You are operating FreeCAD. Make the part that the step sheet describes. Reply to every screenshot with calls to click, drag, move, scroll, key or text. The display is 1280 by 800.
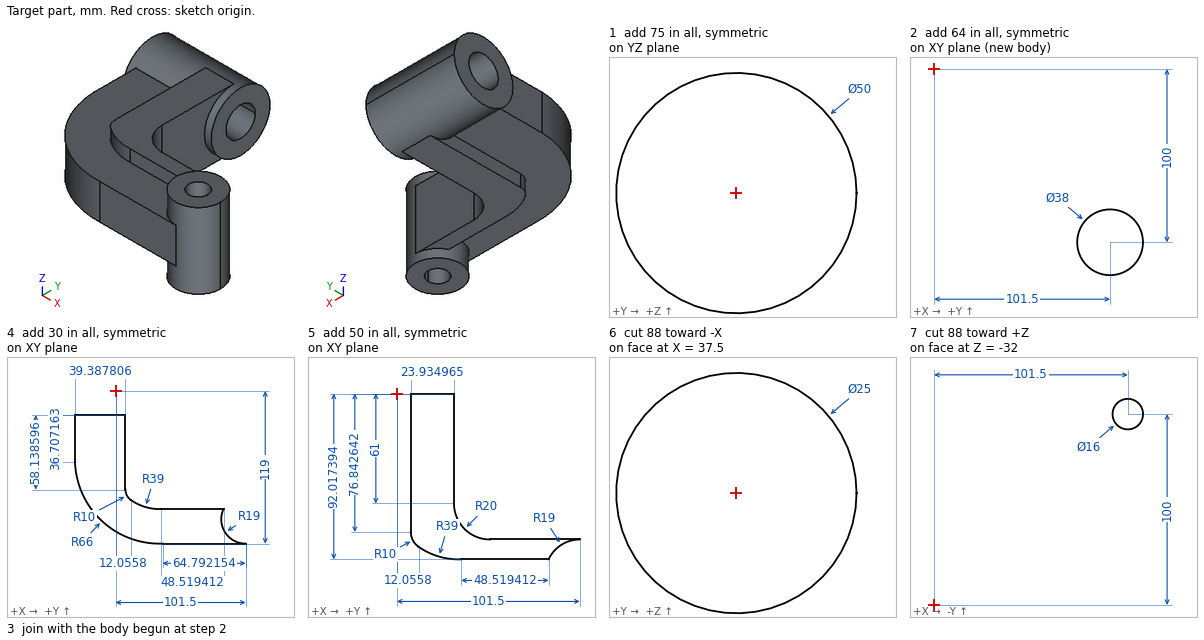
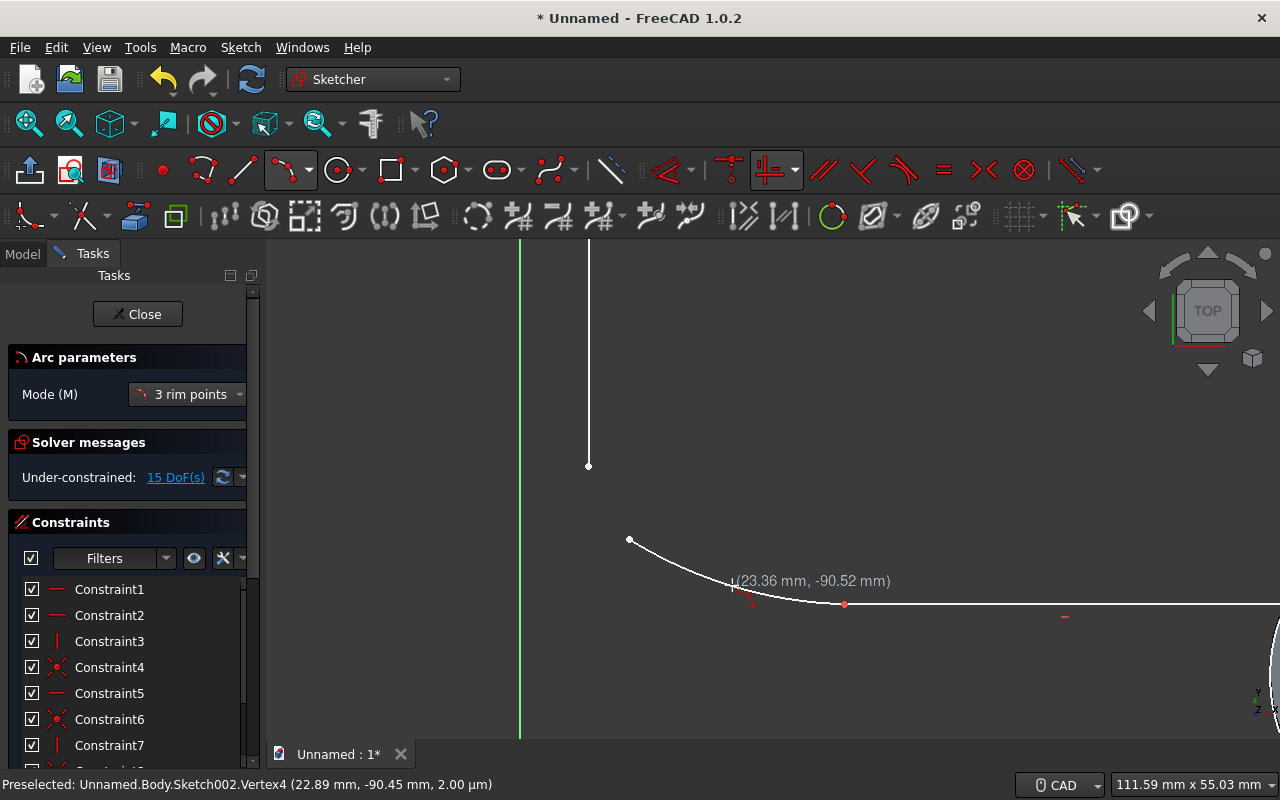
scroll(647, 569, down, 6)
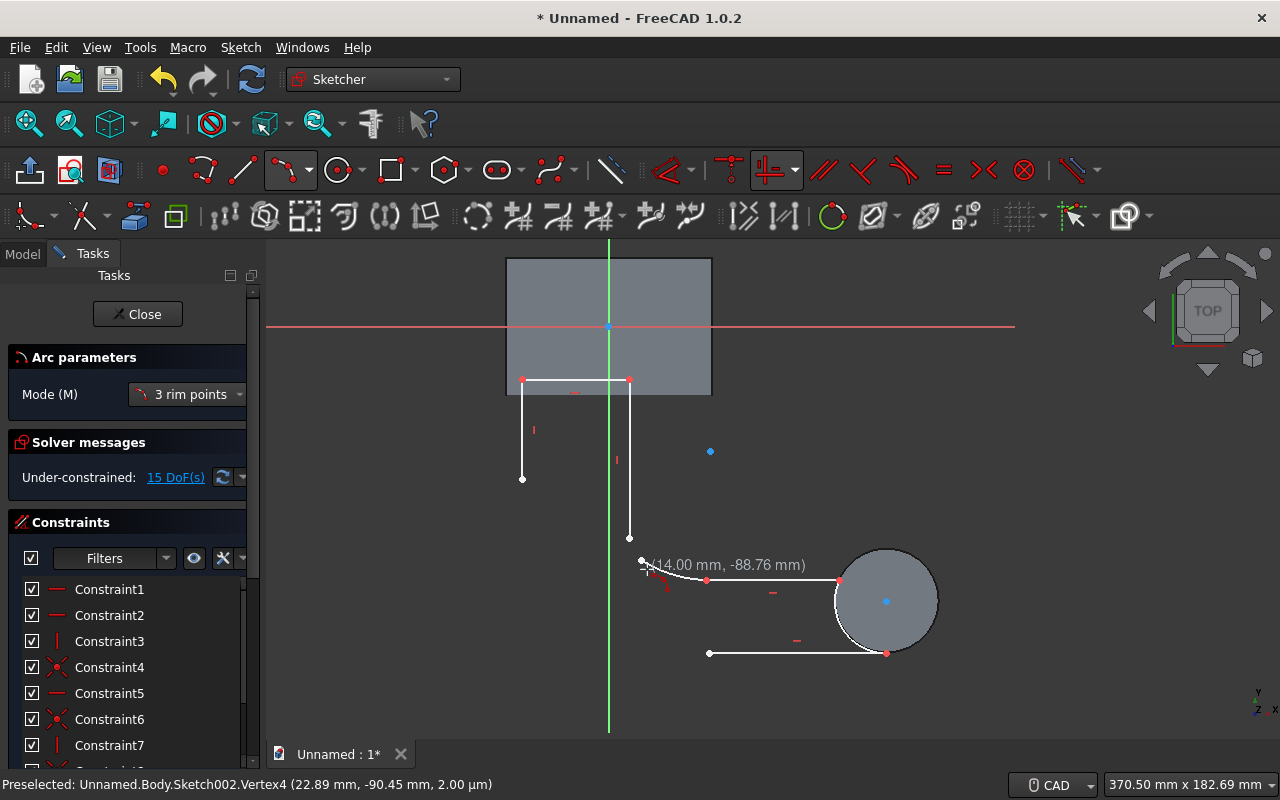
click(642, 561)
click(630, 539)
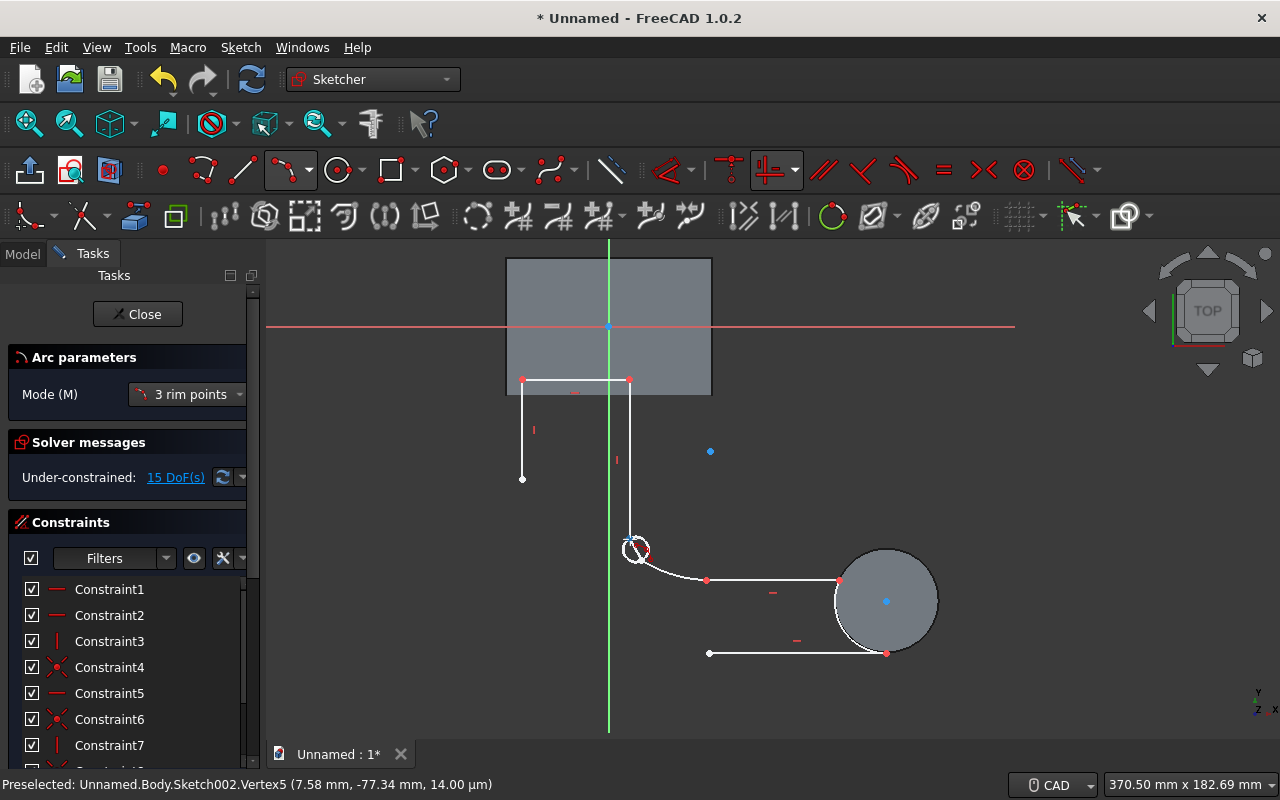
scroll(633, 550, up, 9)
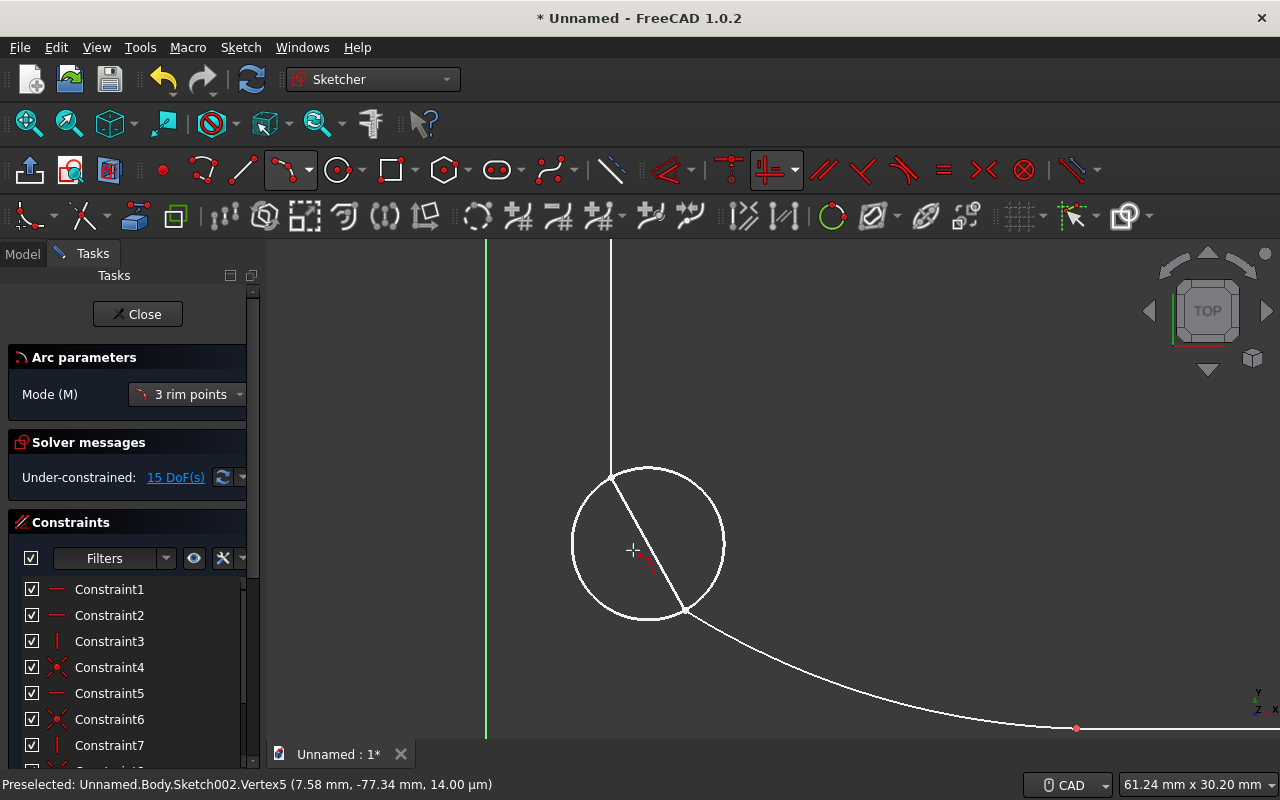
click(633, 546)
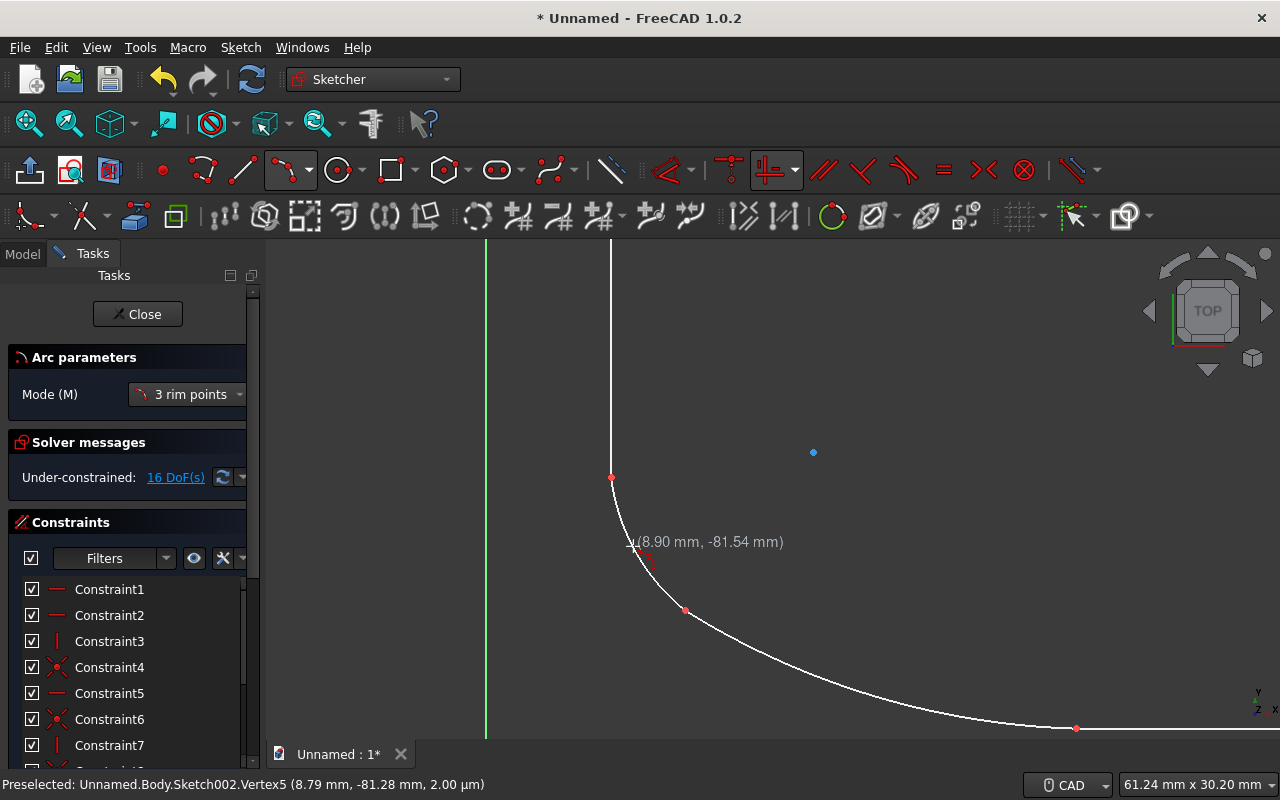
scroll(633, 550, down, 9)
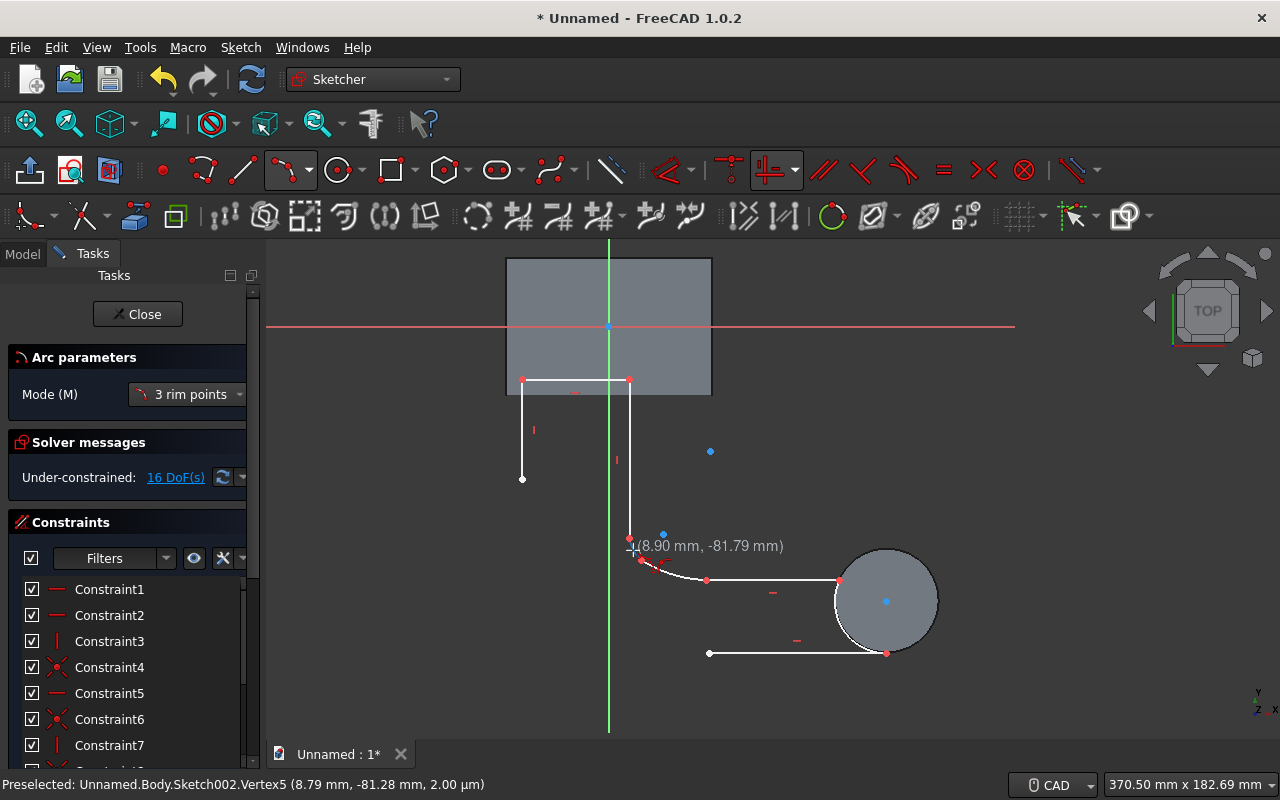
click(522, 480)
click(709, 653)
click(580, 604)
key(Escape)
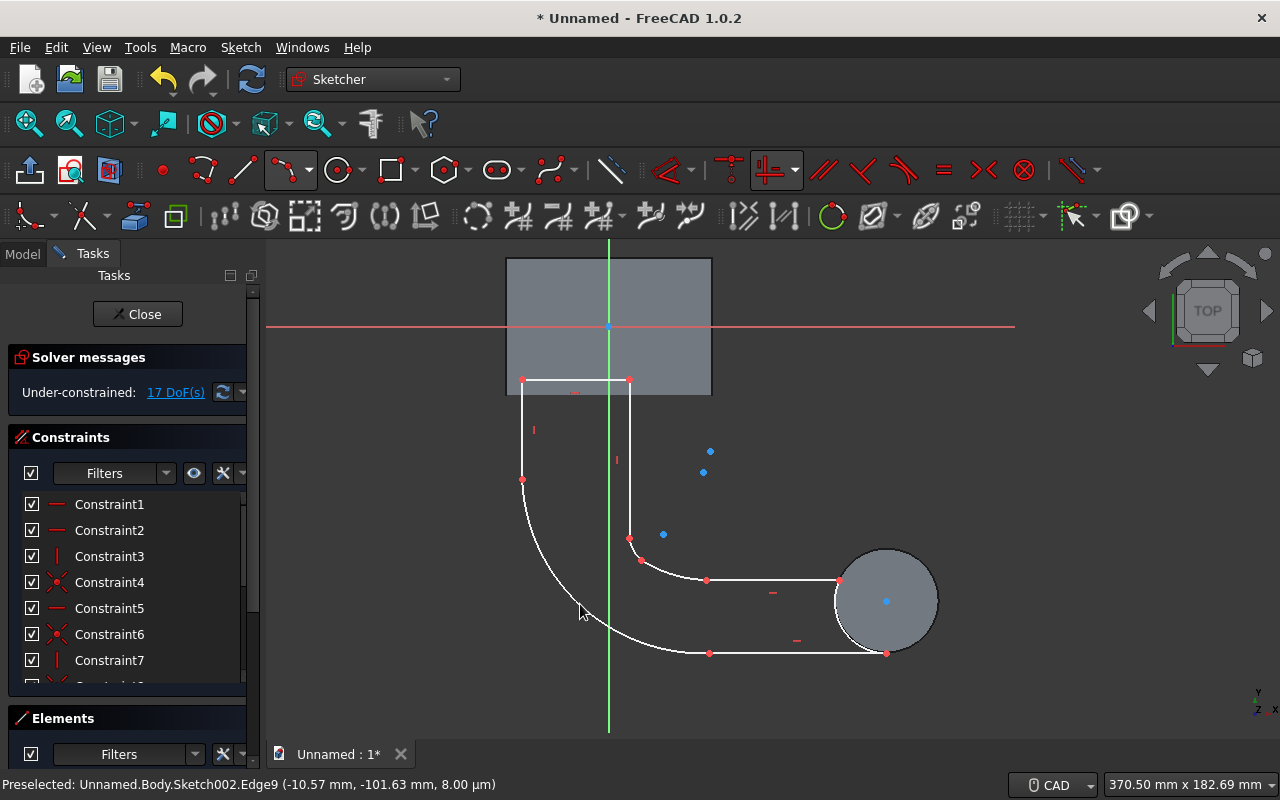
click(762, 653)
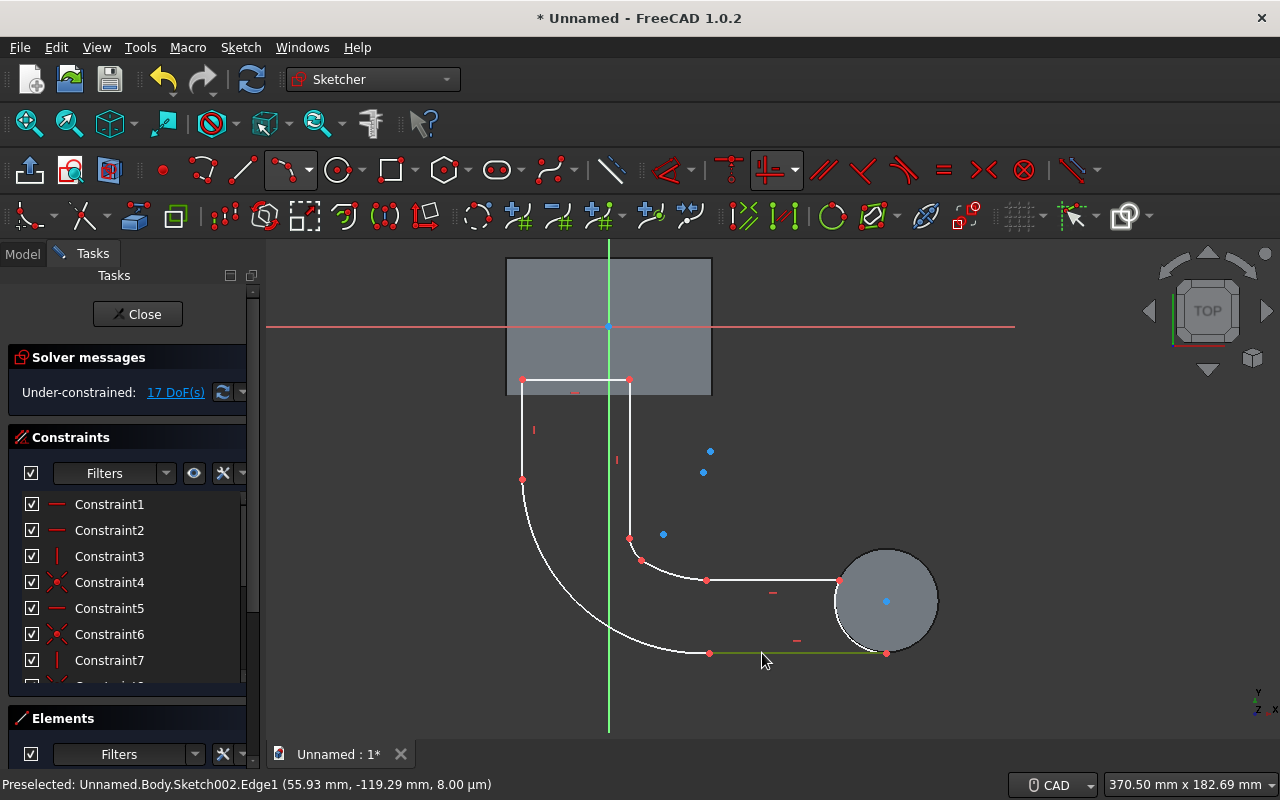
click(836, 610)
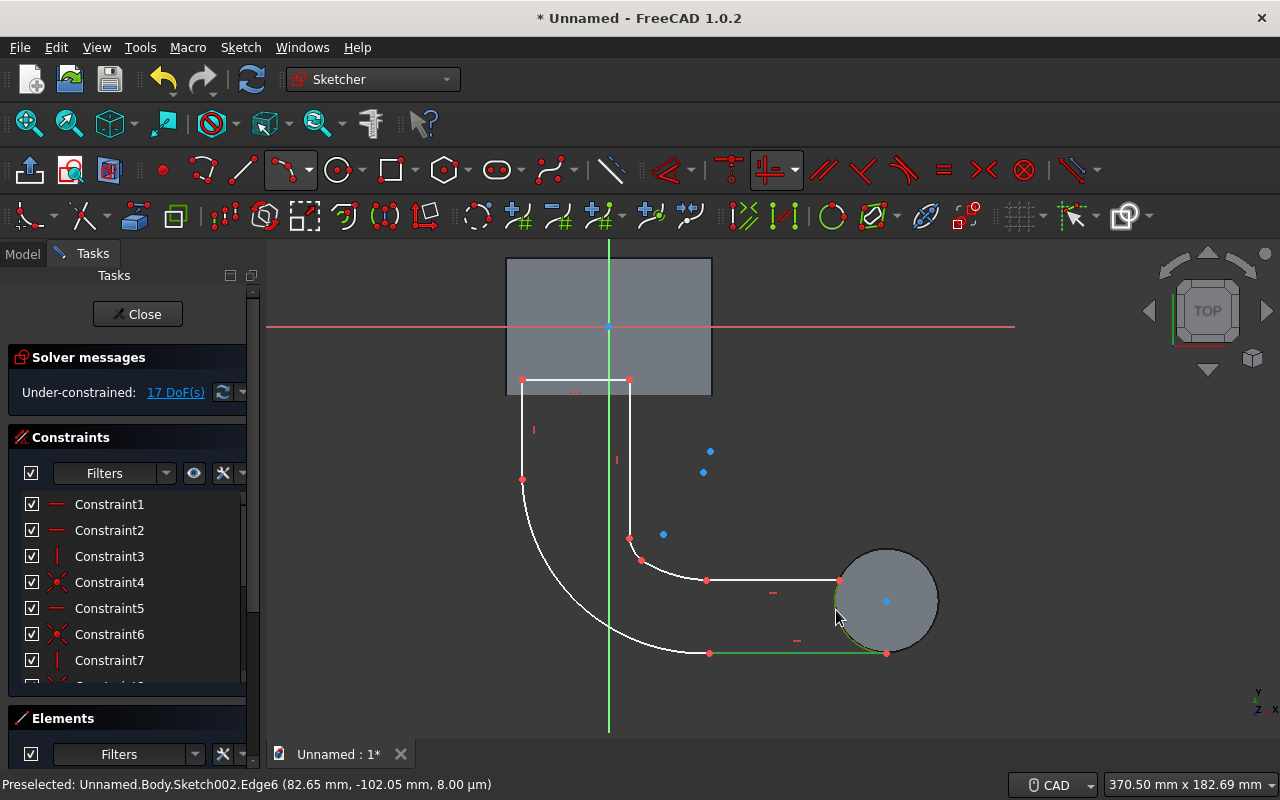
click(904, 170)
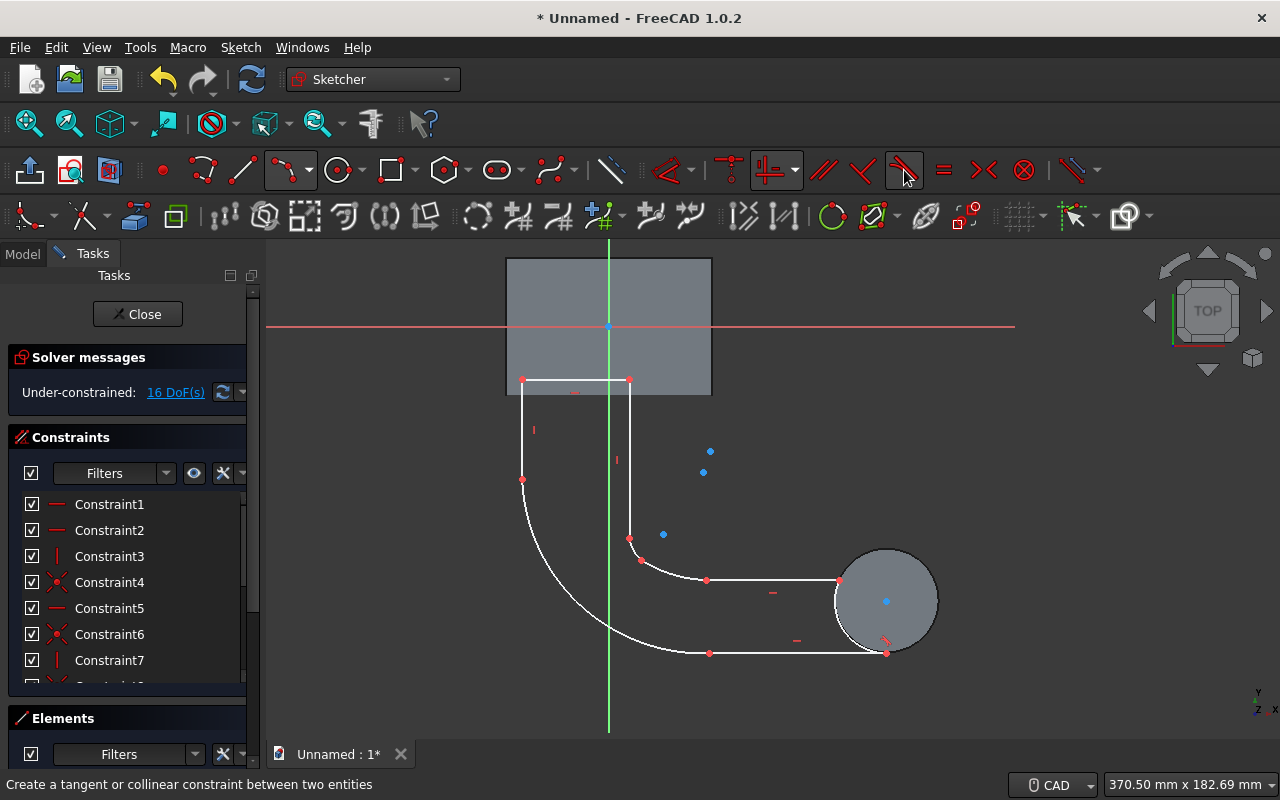
click(630, 491)